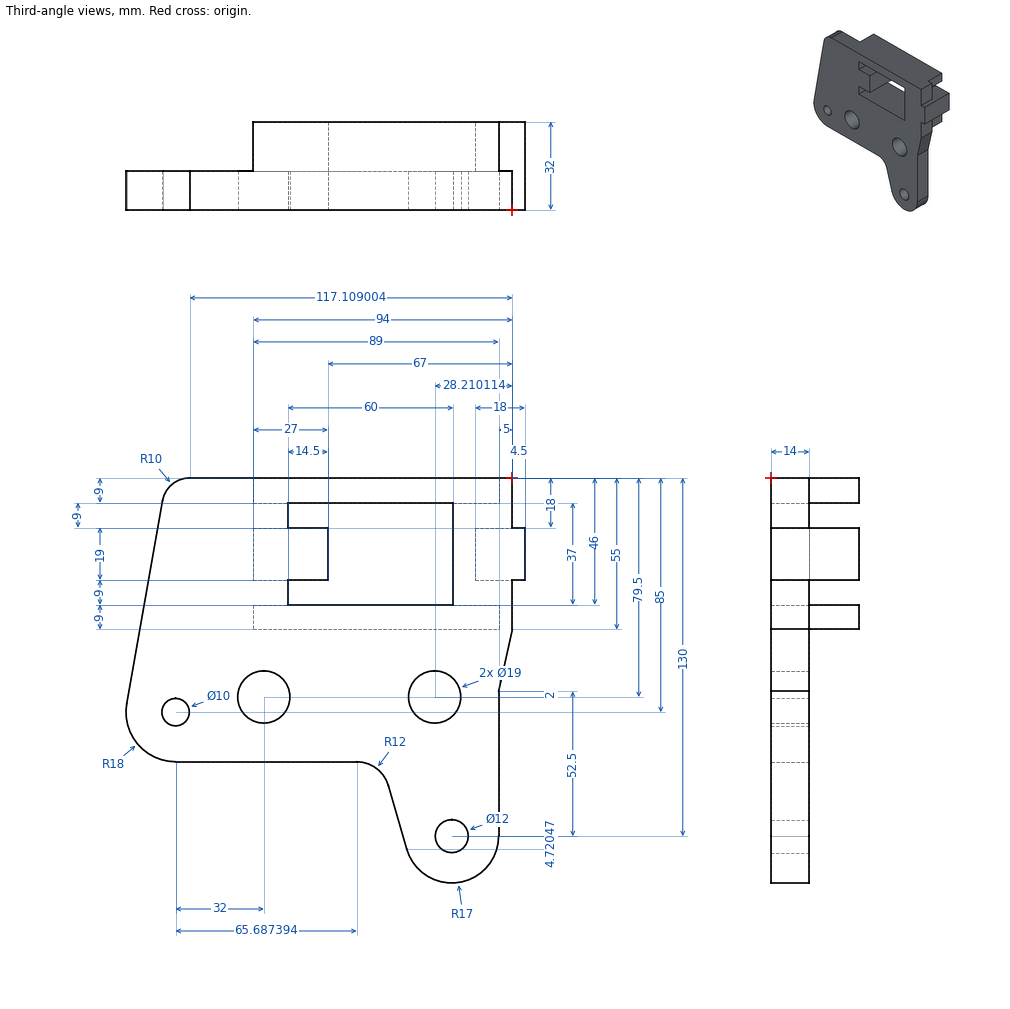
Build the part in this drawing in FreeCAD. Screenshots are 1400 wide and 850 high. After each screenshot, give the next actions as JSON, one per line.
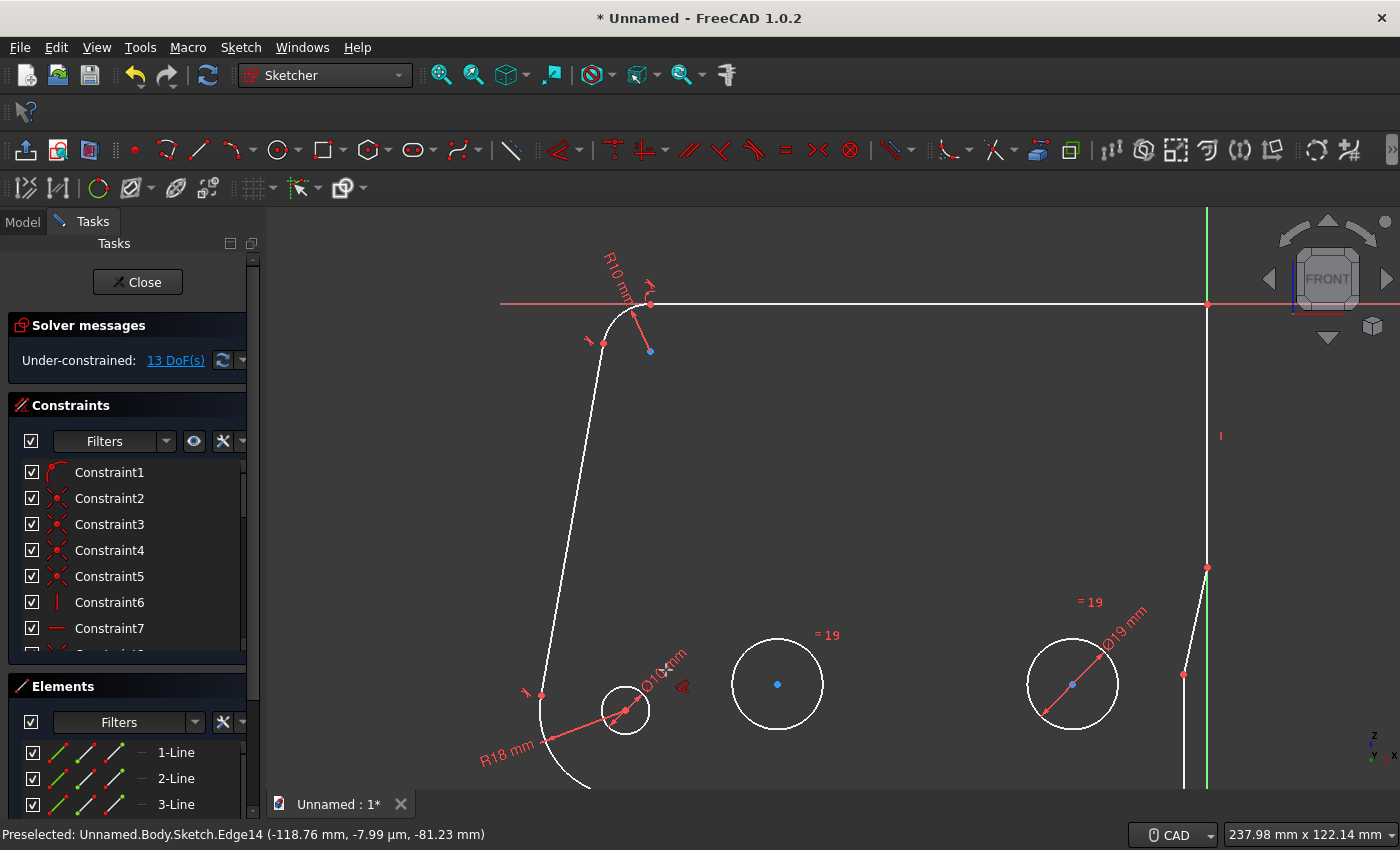
{"action": "scroll", "coordinate": [631, 308], "scroll_direction": "down", "scroll_amount": 3}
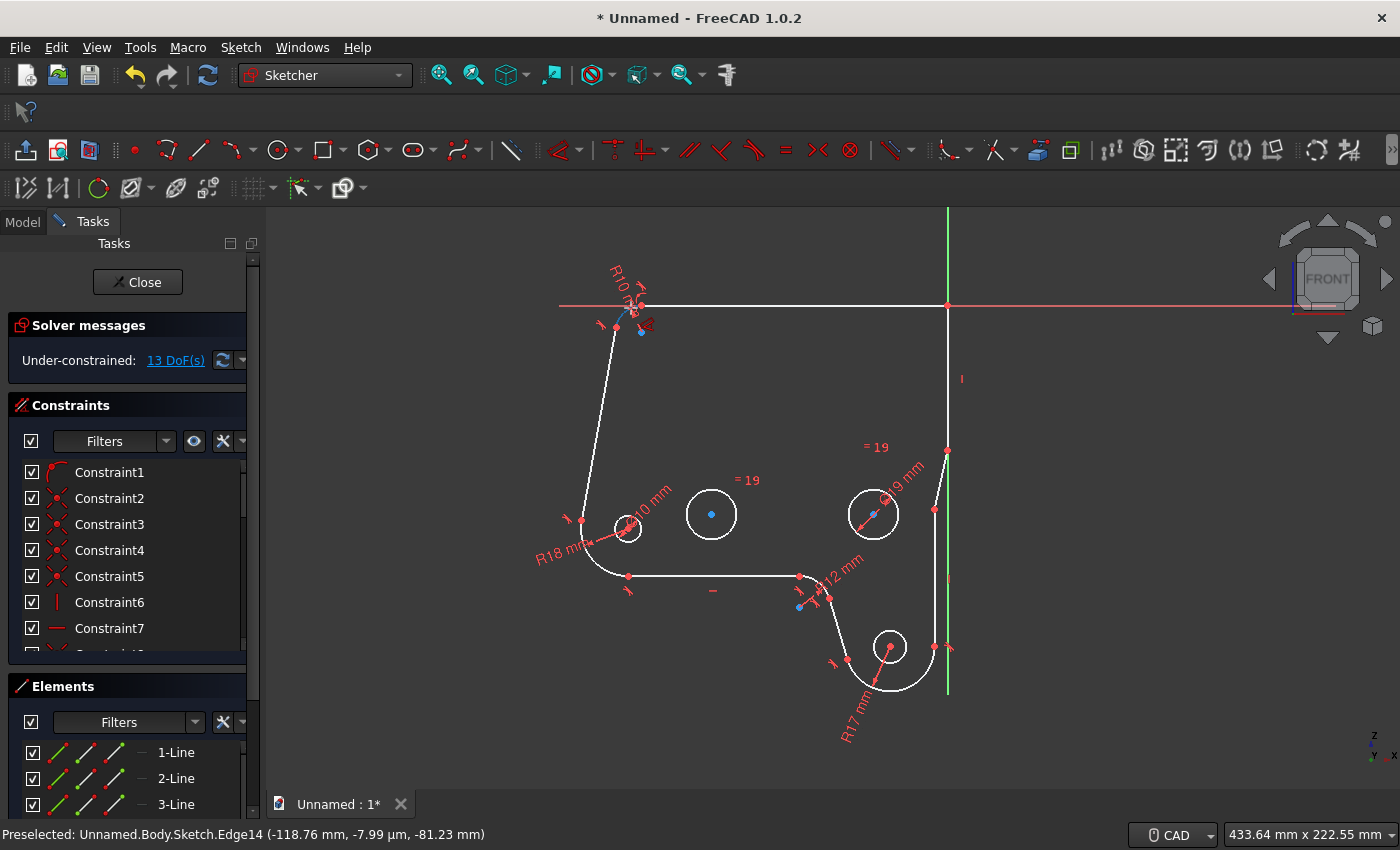
{"action": "scroll", "coordinate": [901, 635], "scroll_direction": "up", "scroll_amount": 2}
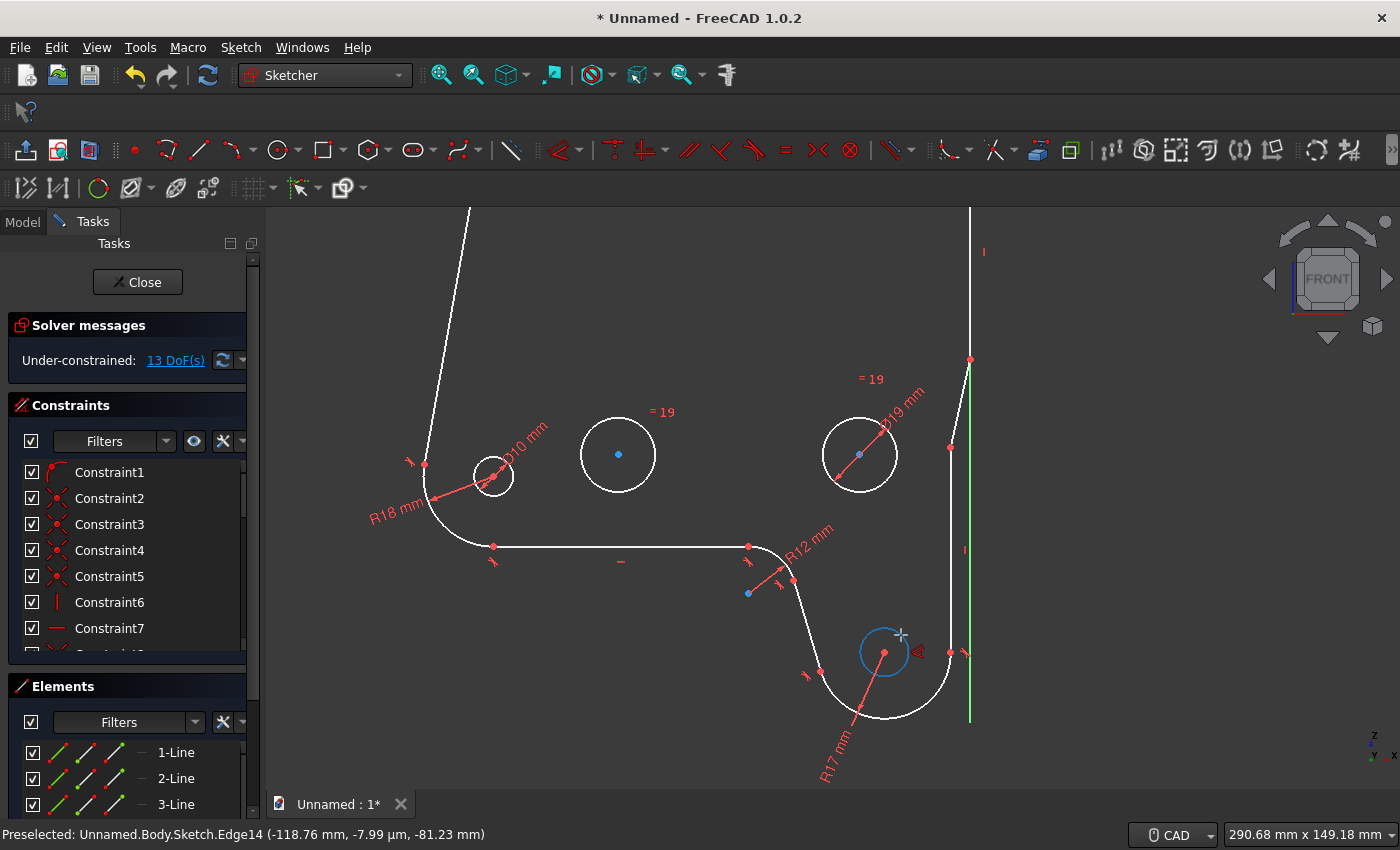
{"action": "left_click", "coordinate": [901, 635]}
{"action": "left_click", "coordinate": [923, 612]}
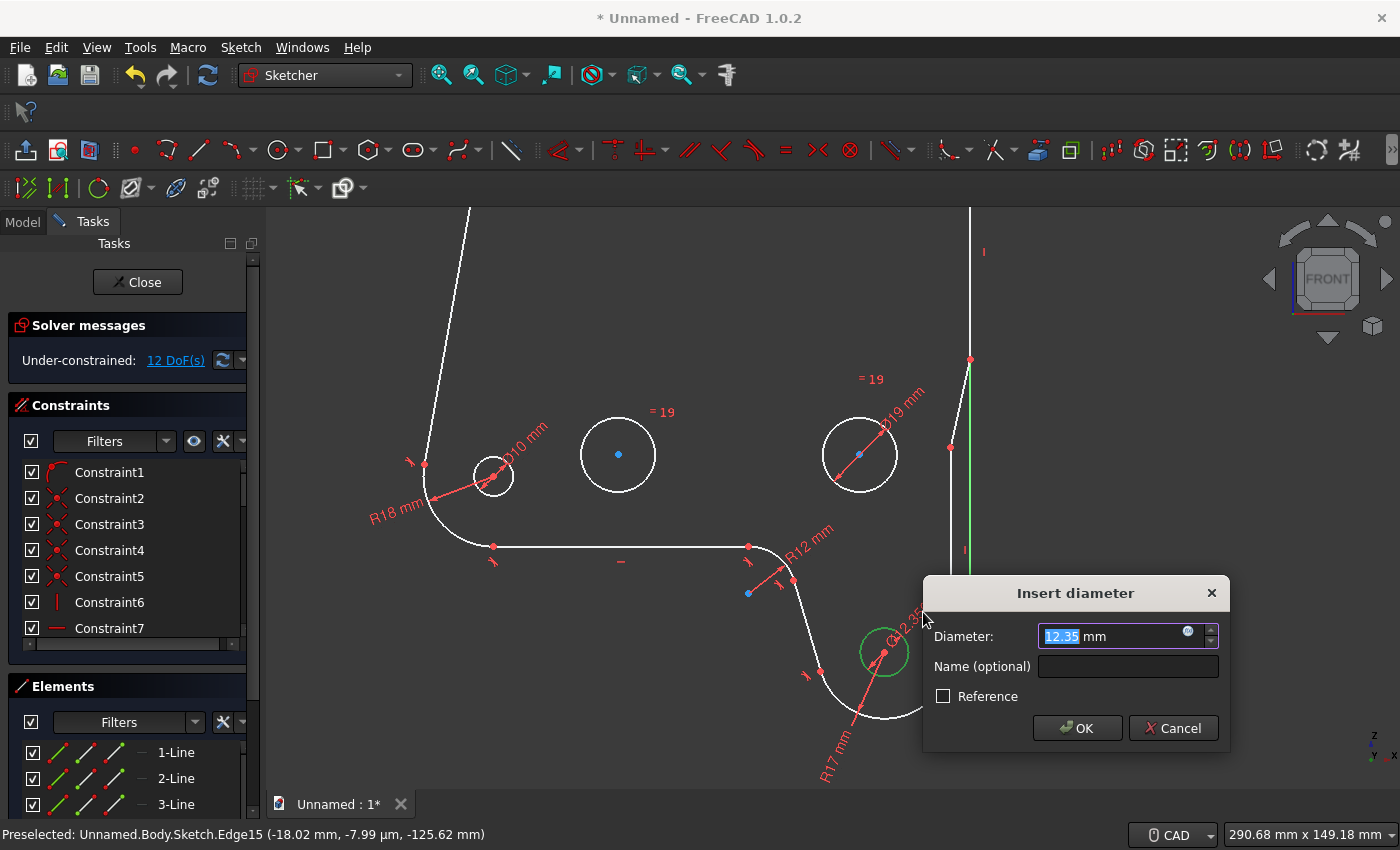
{"action": "type", "text": "12"}
{"action": "key", "text": "Return"}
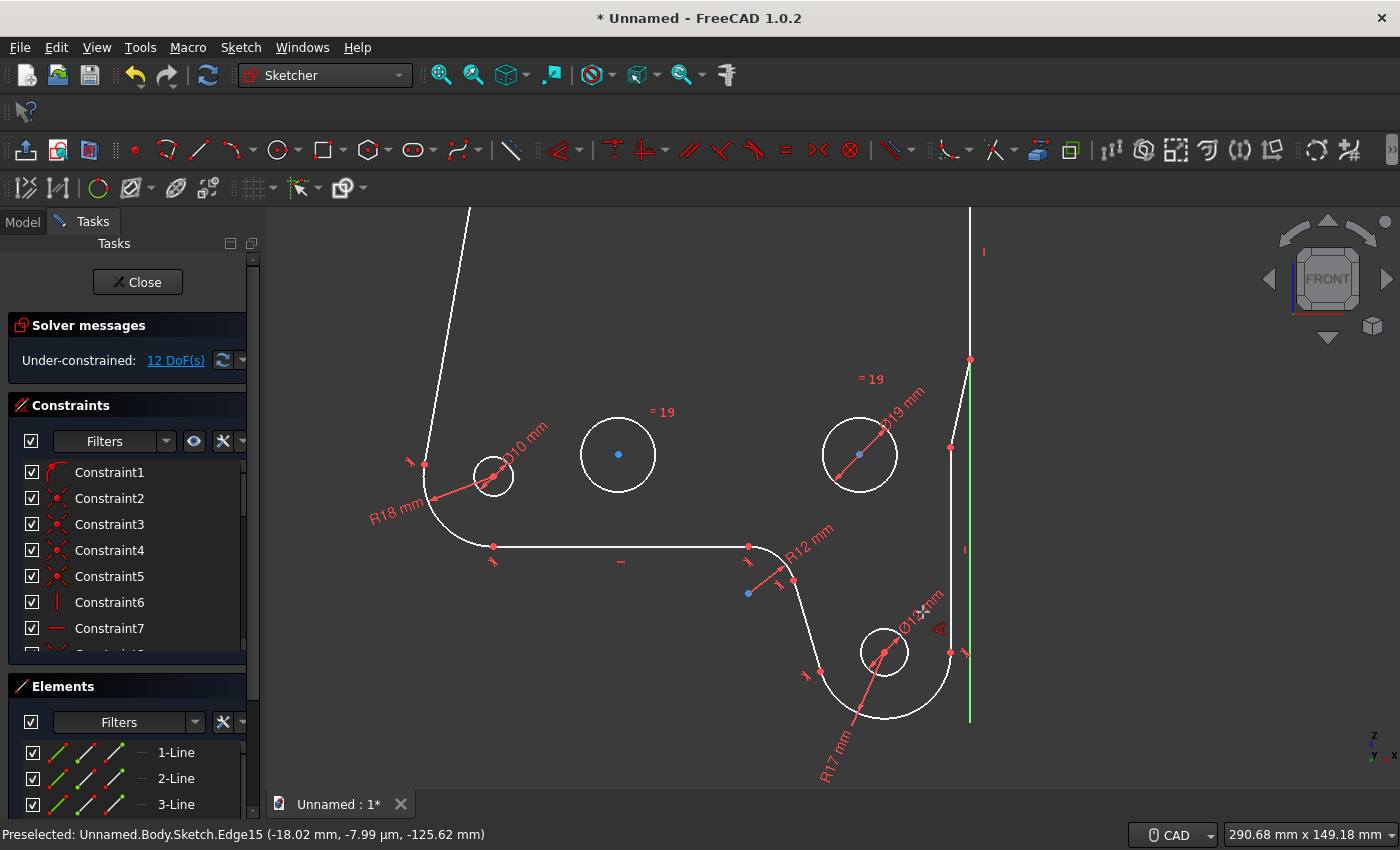
{"action": "left_click", "coordinate": [970, 295]}
{"action": "left_click", "coordinate": [1004, 297]}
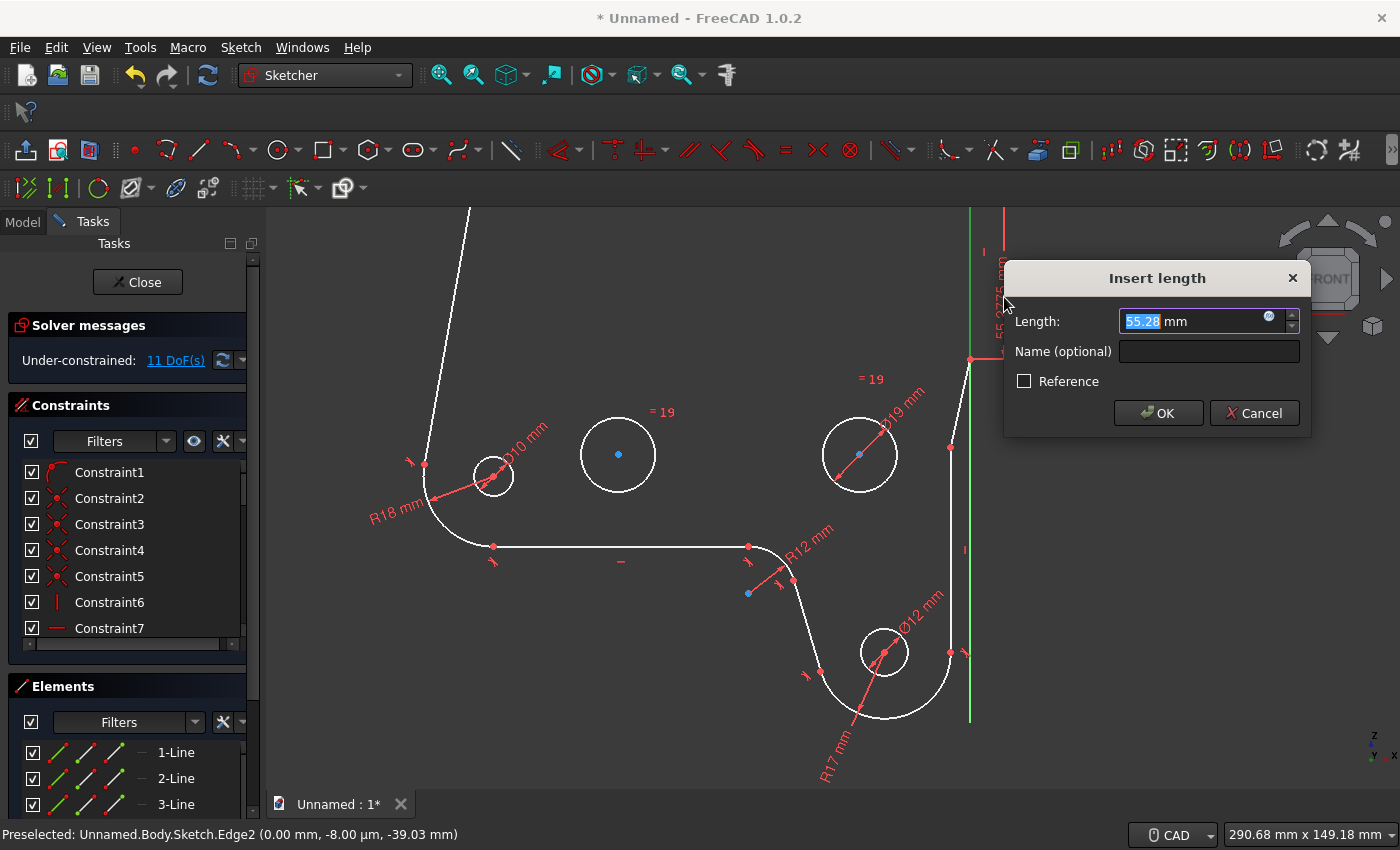
{"action": "type", "text": "55"}
{"action": "key", "text": "Return"}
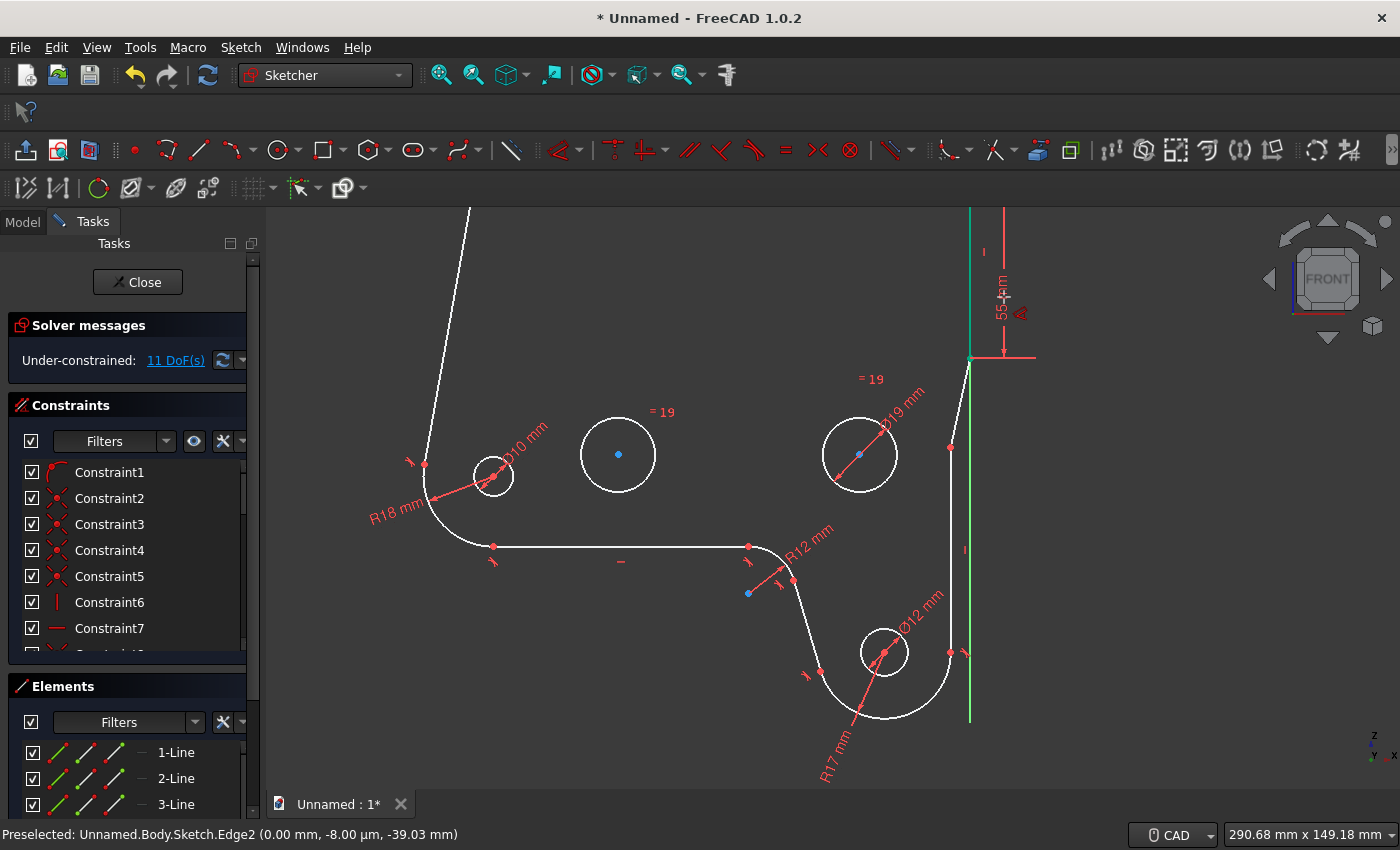
{"action": "scroll", "coordinate": [951, 447], "scroll_direction": "up", "scroll_amount": 4}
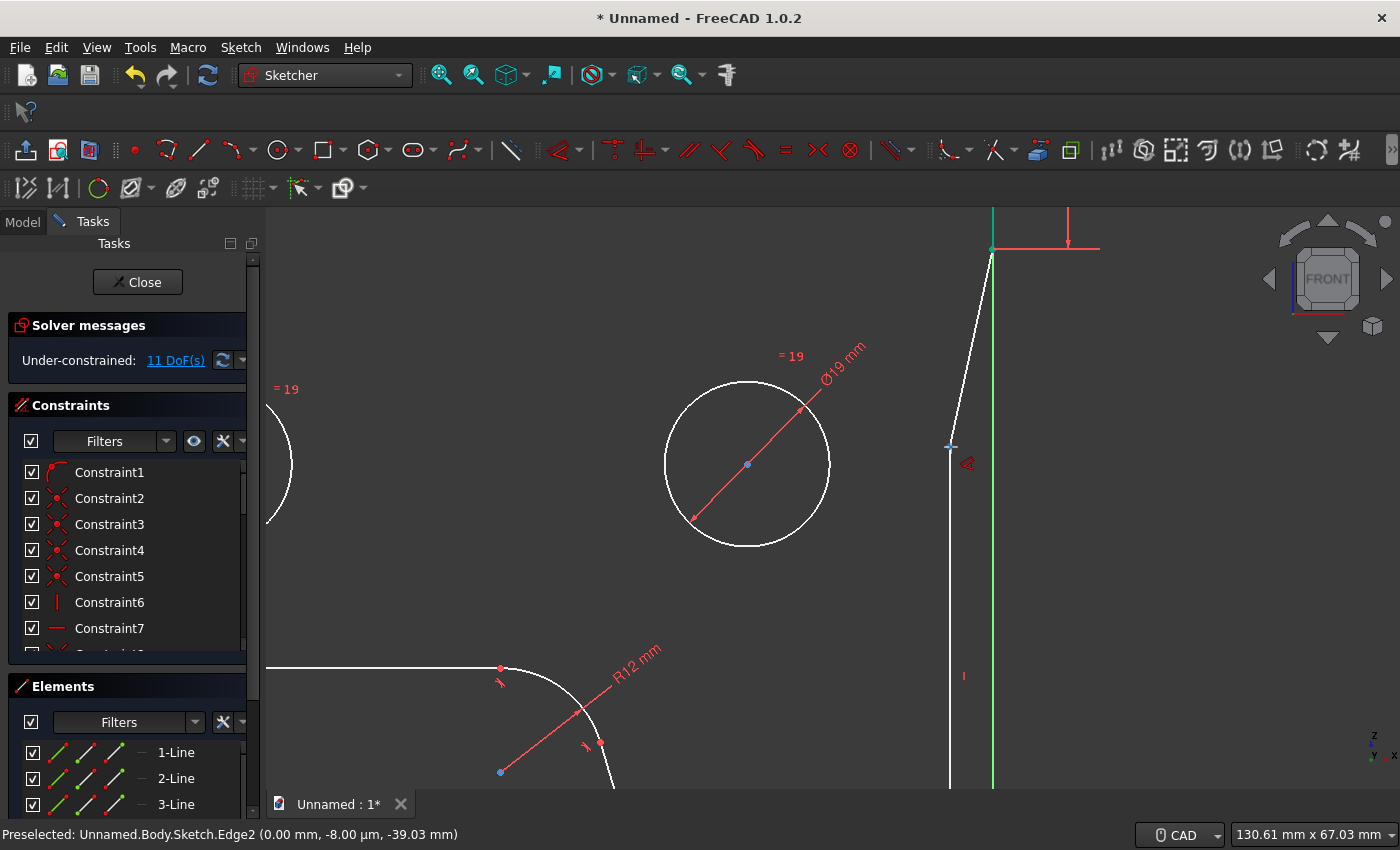
{"action": "left_click", "coordinate": [950, 447]}
{"action": "left_click", "coordinate": [971, 481]}